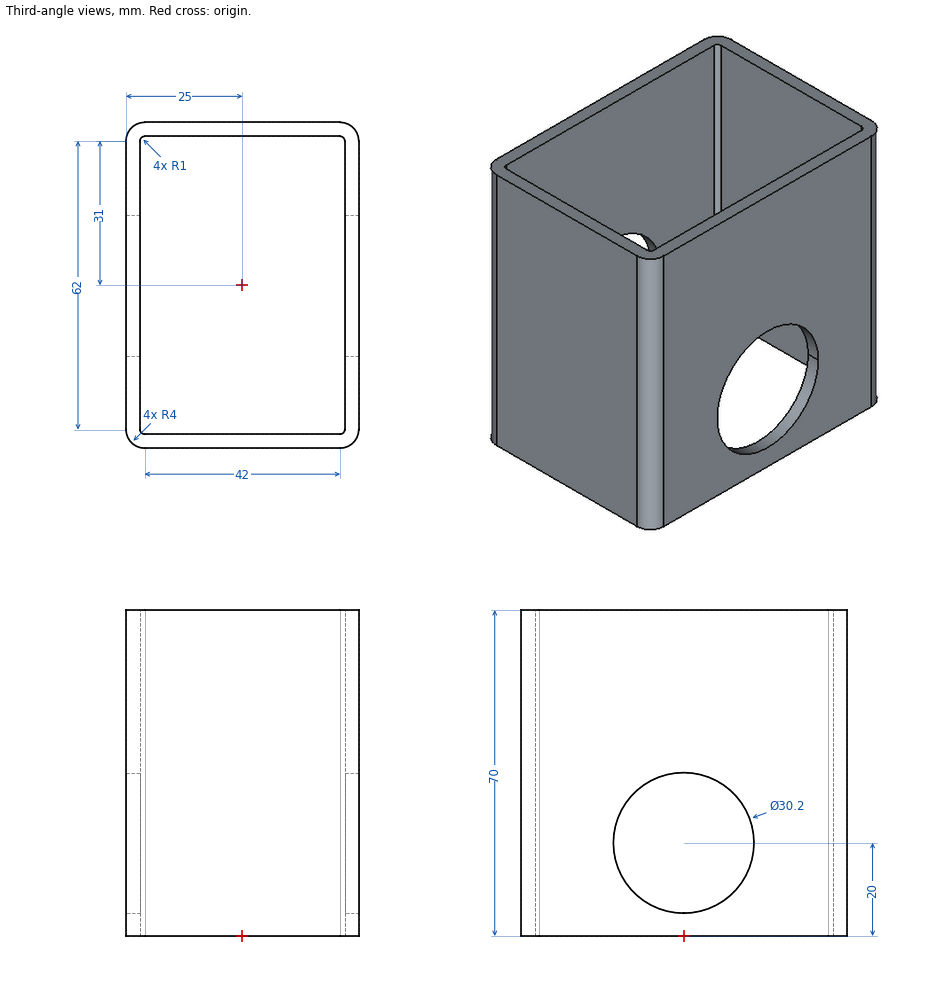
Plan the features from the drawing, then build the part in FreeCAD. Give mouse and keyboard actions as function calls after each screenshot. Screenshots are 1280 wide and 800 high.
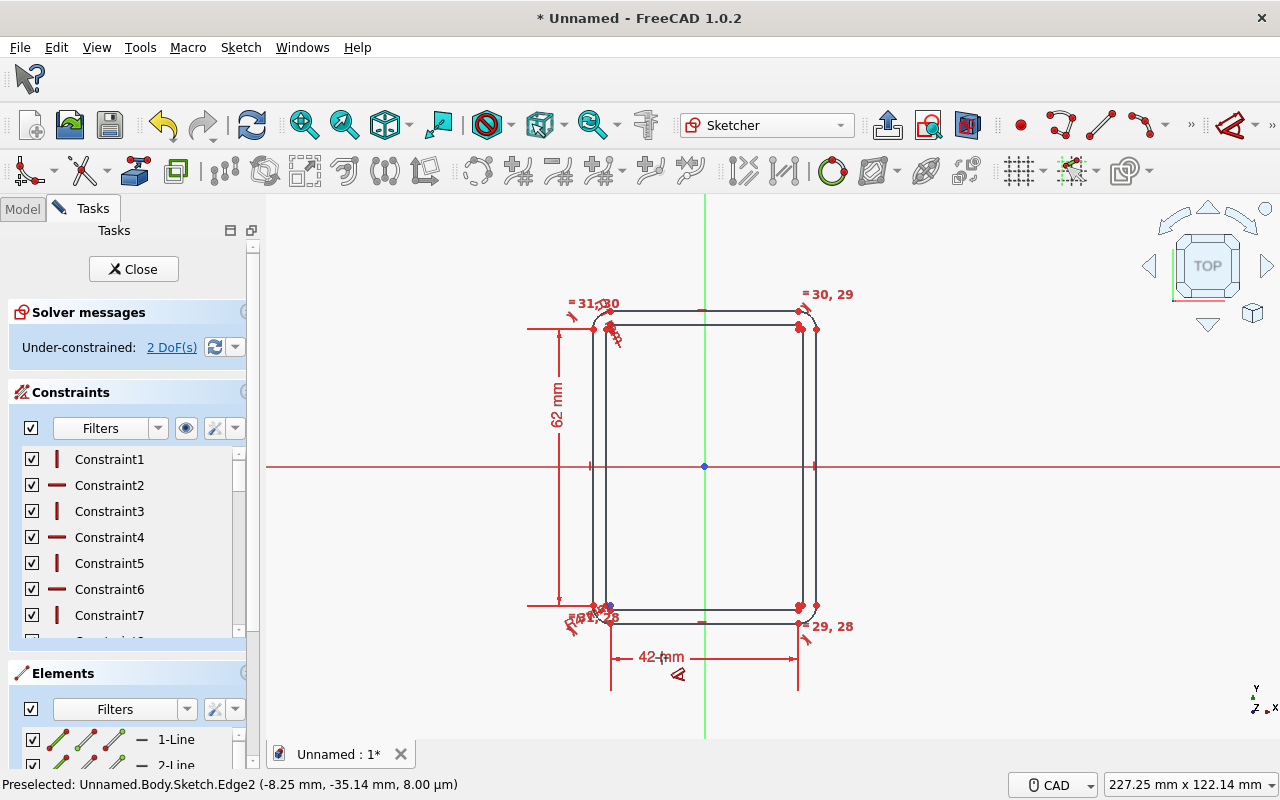
click(593, 329)
click(649, 295)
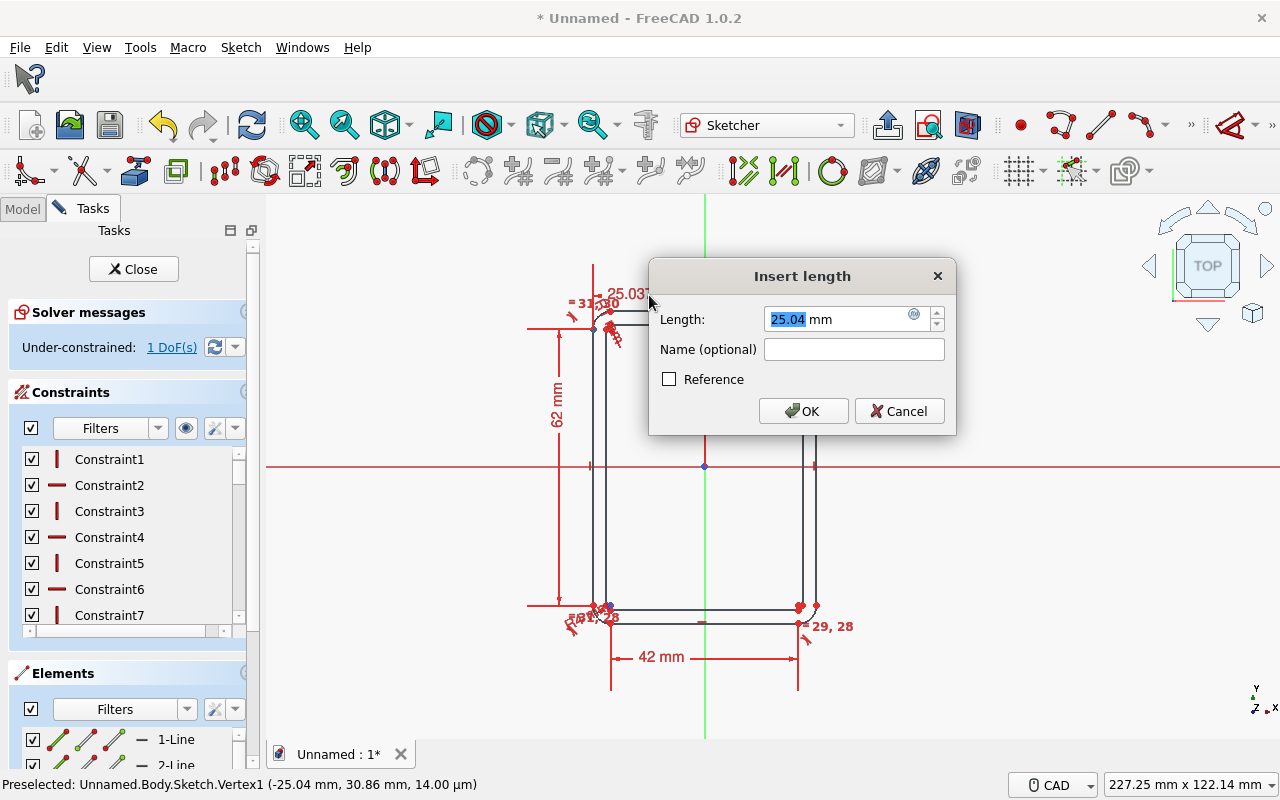
text(25)
key(Return)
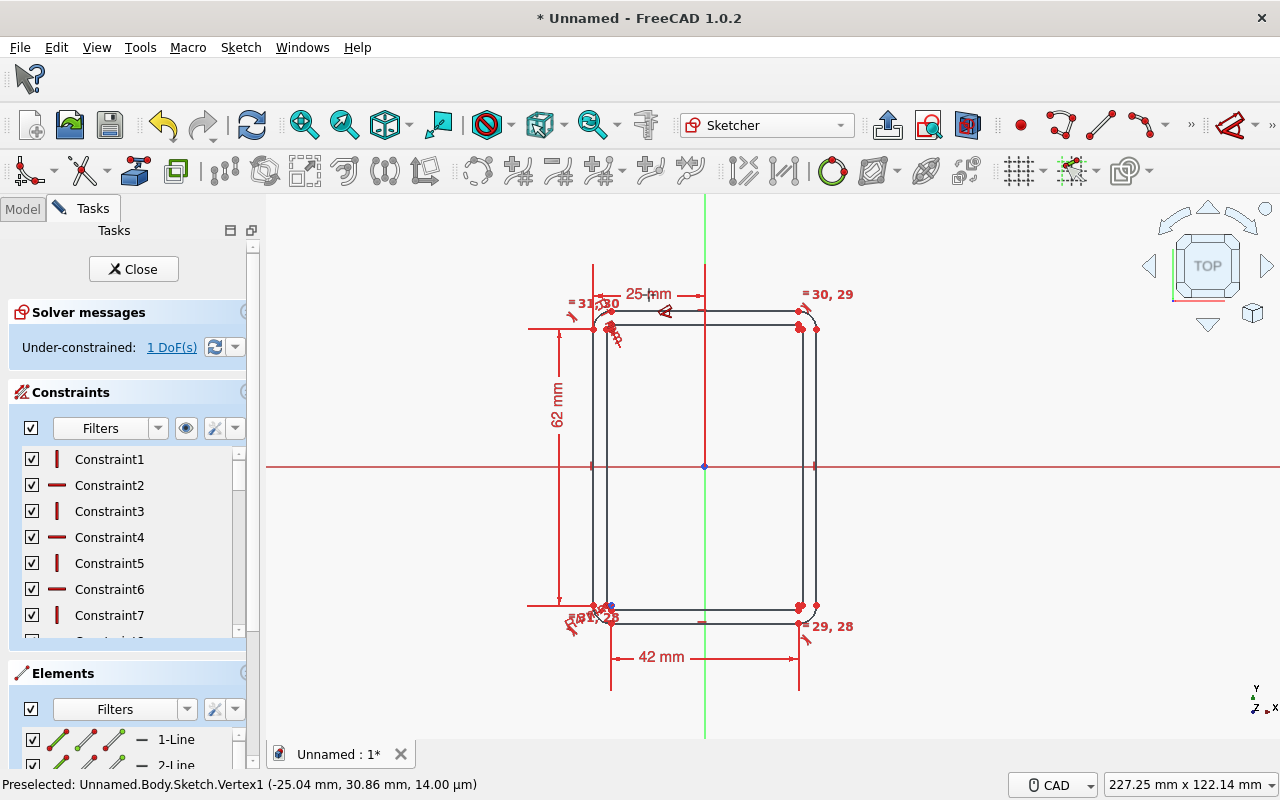
click(593, 329)
click(559, 366)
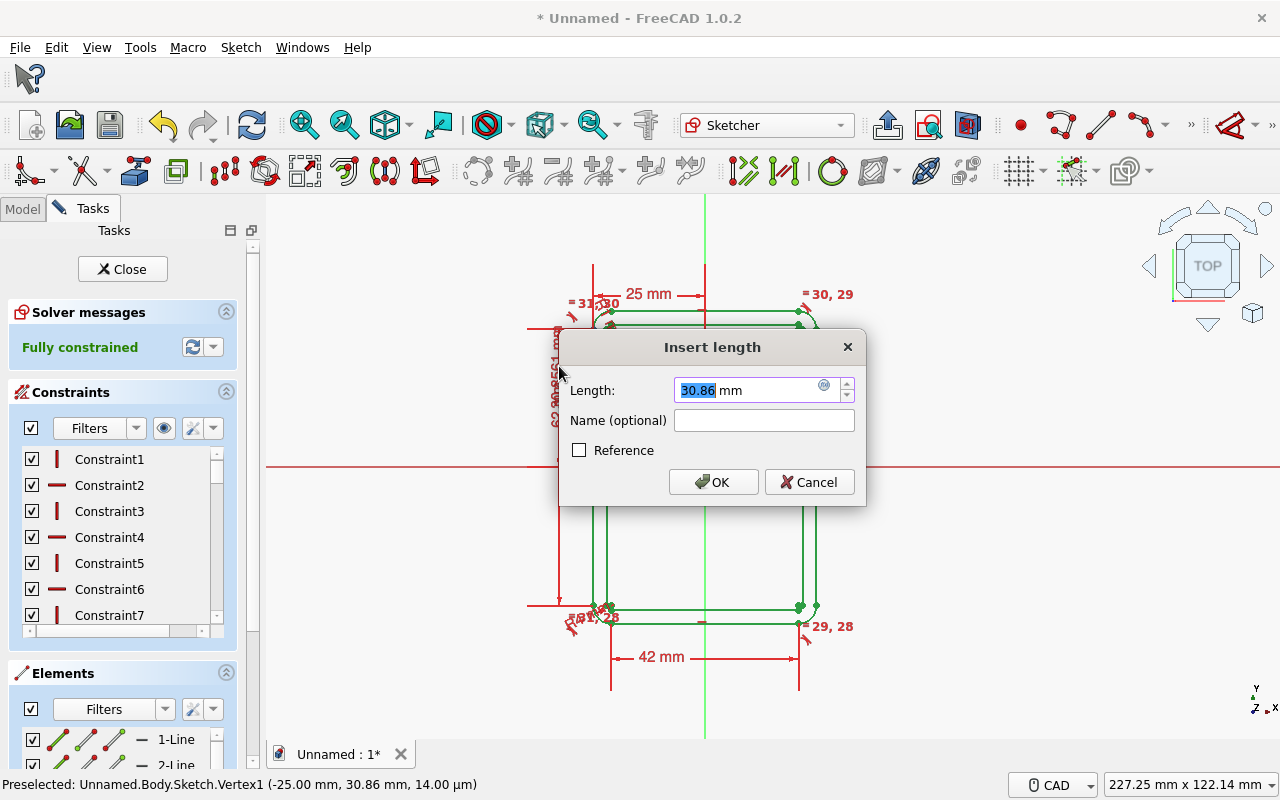
text(31)
key(Return)
key(Escape)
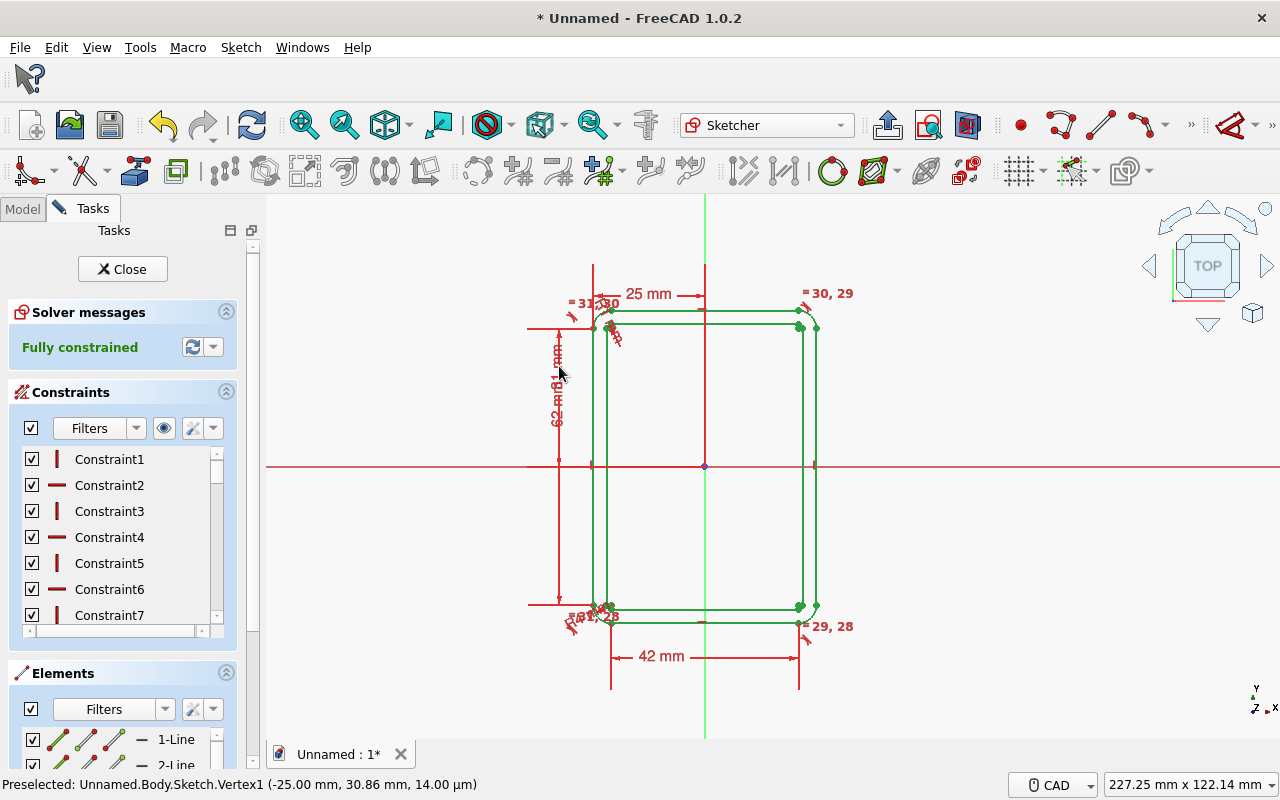
click(123, 269)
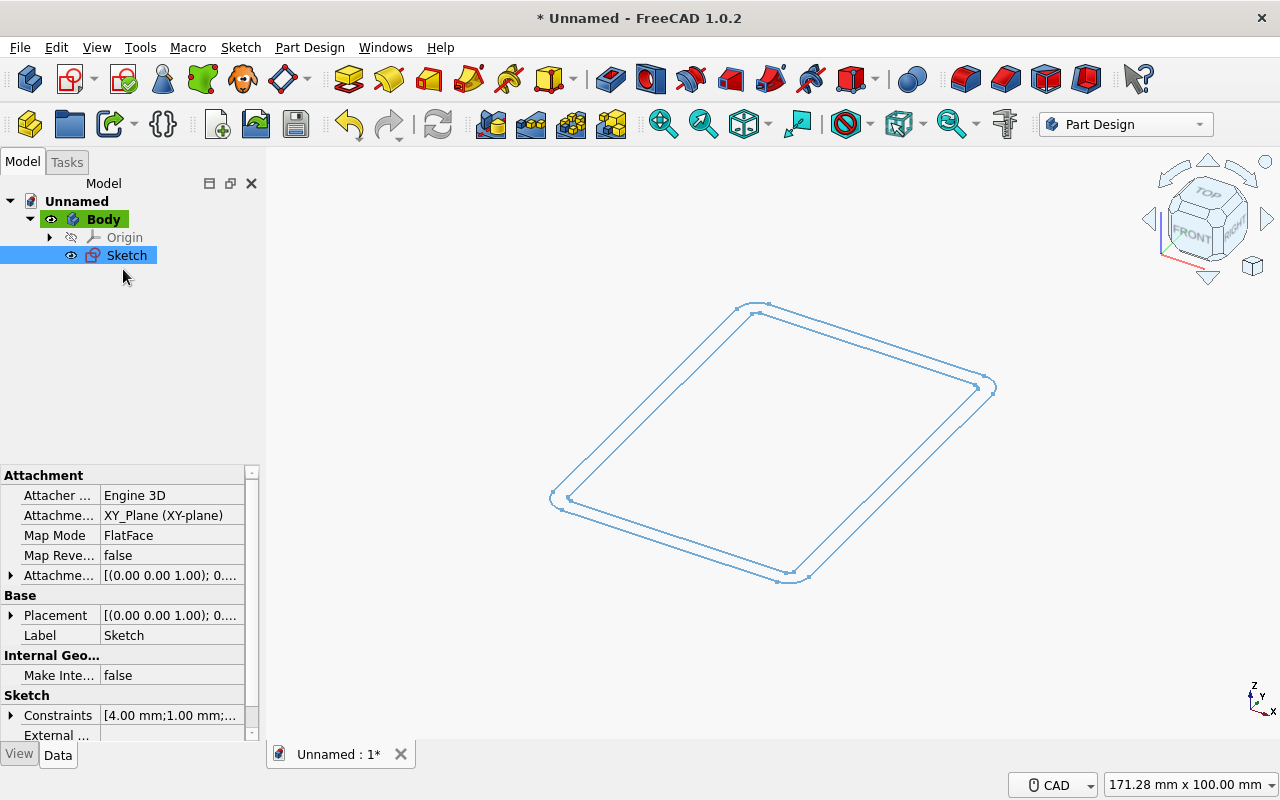
click(350, 80)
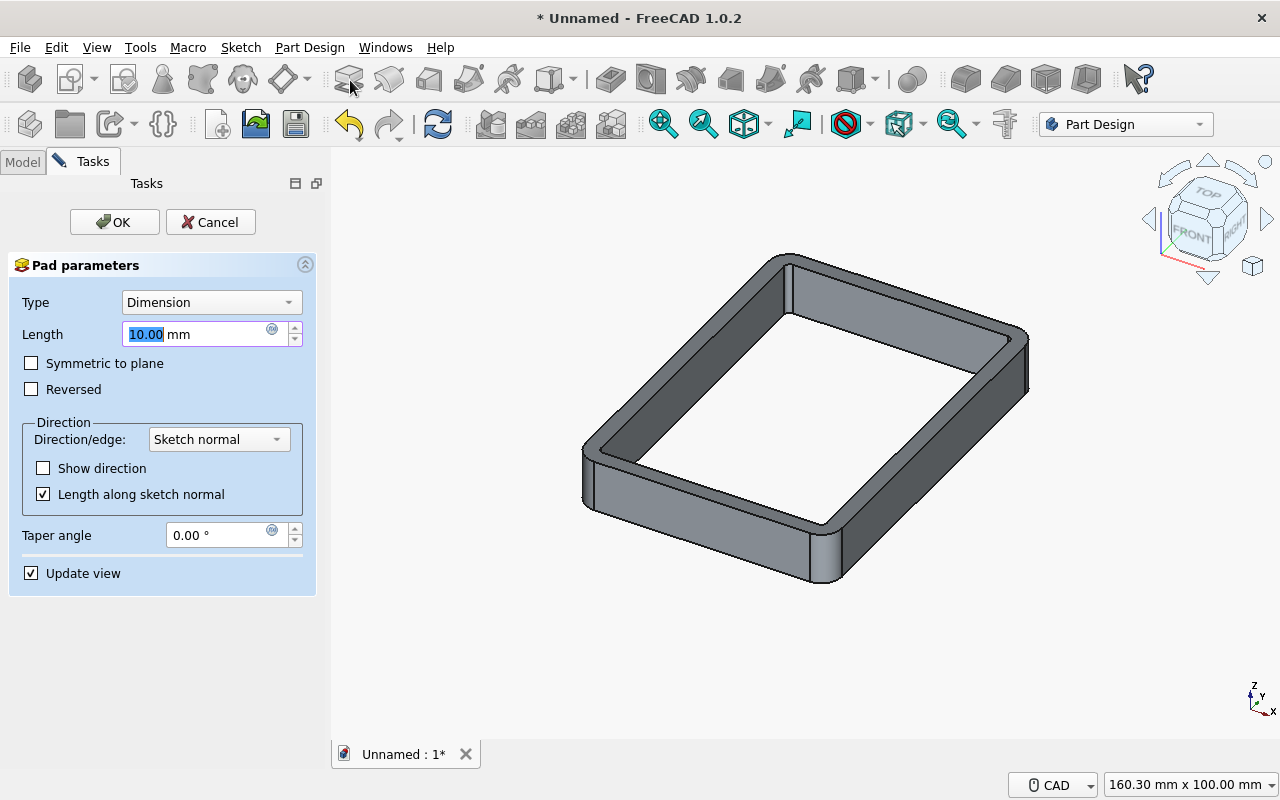
text(70)
key(Tab)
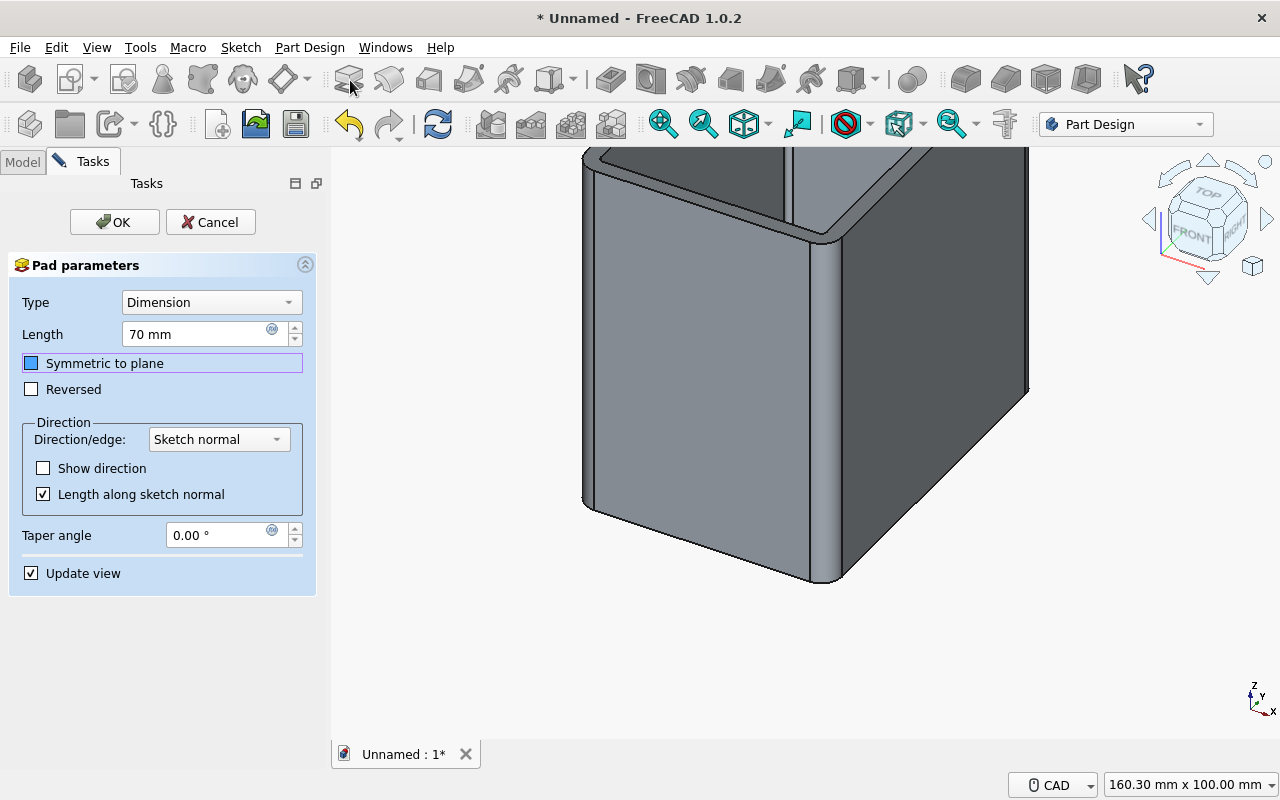
click(115, 222)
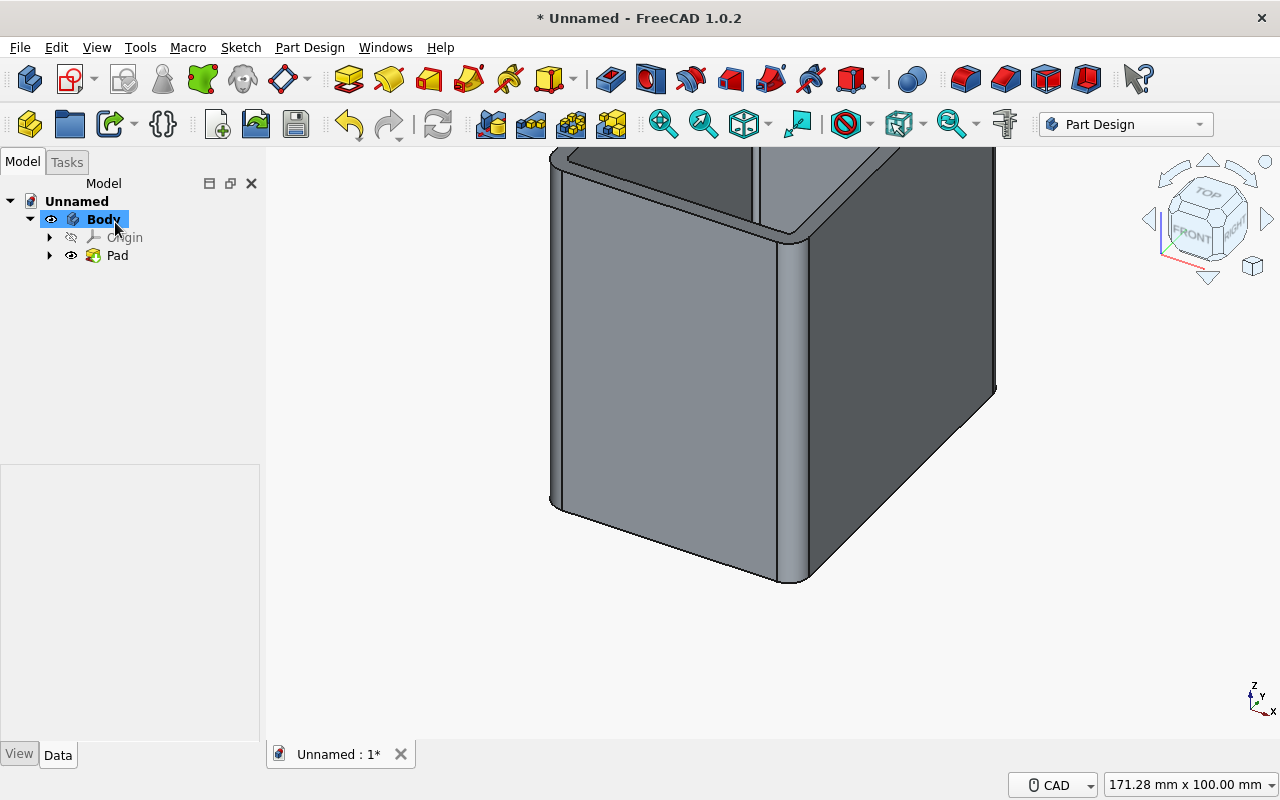
click(664, 124)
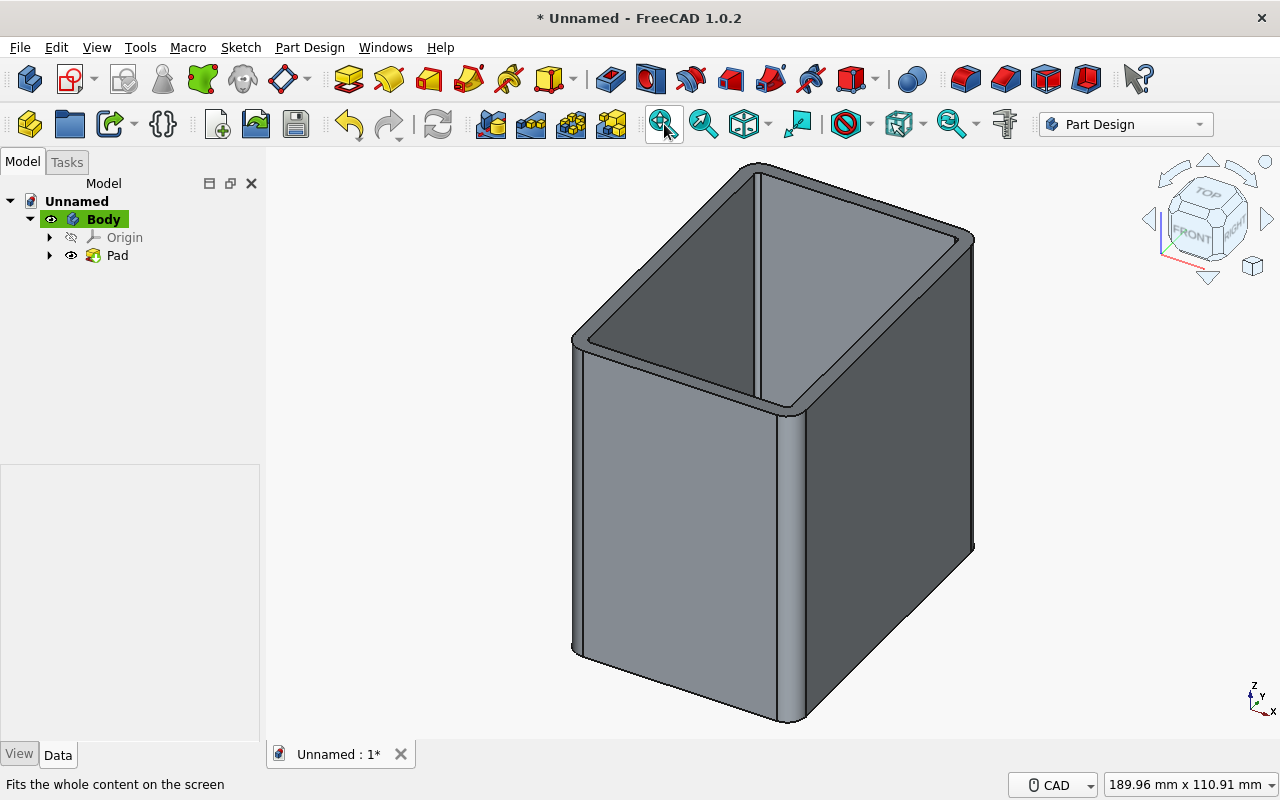
click(889, 480)